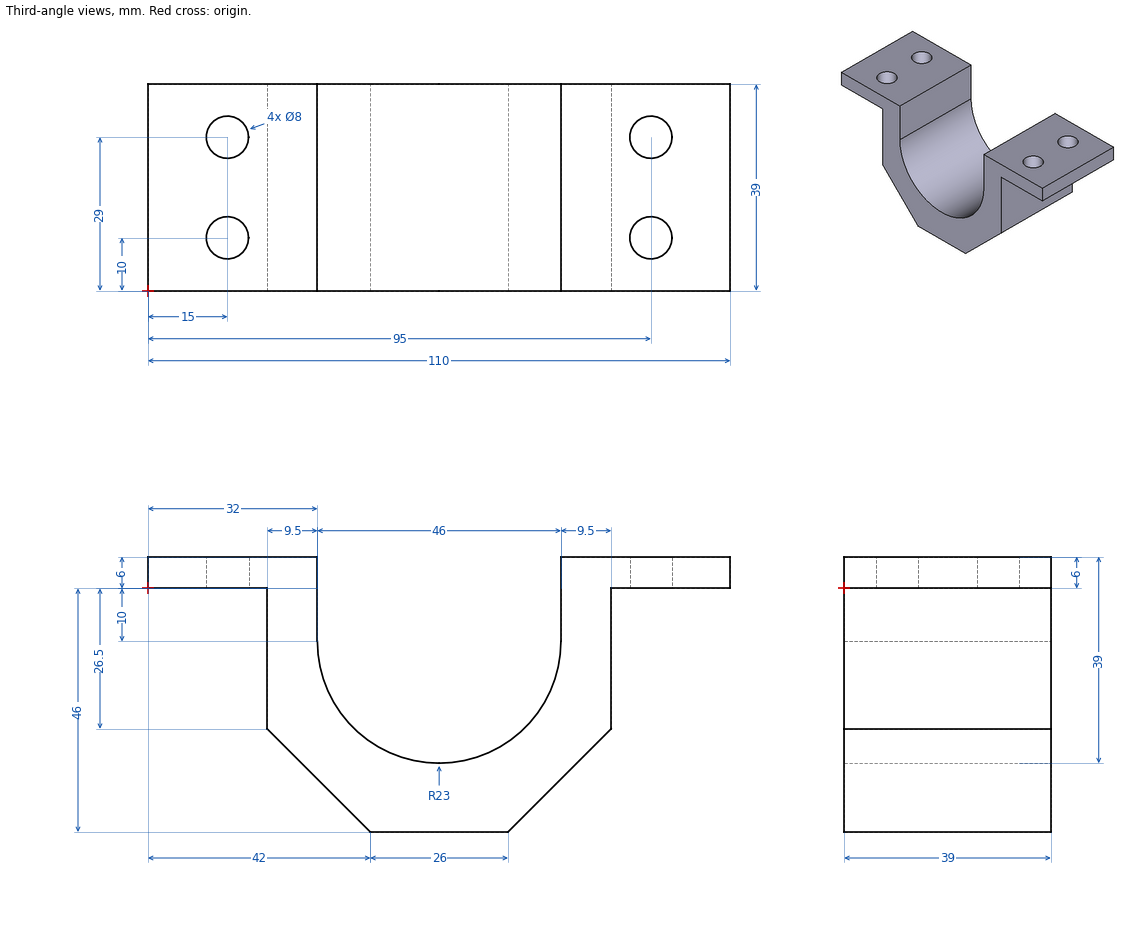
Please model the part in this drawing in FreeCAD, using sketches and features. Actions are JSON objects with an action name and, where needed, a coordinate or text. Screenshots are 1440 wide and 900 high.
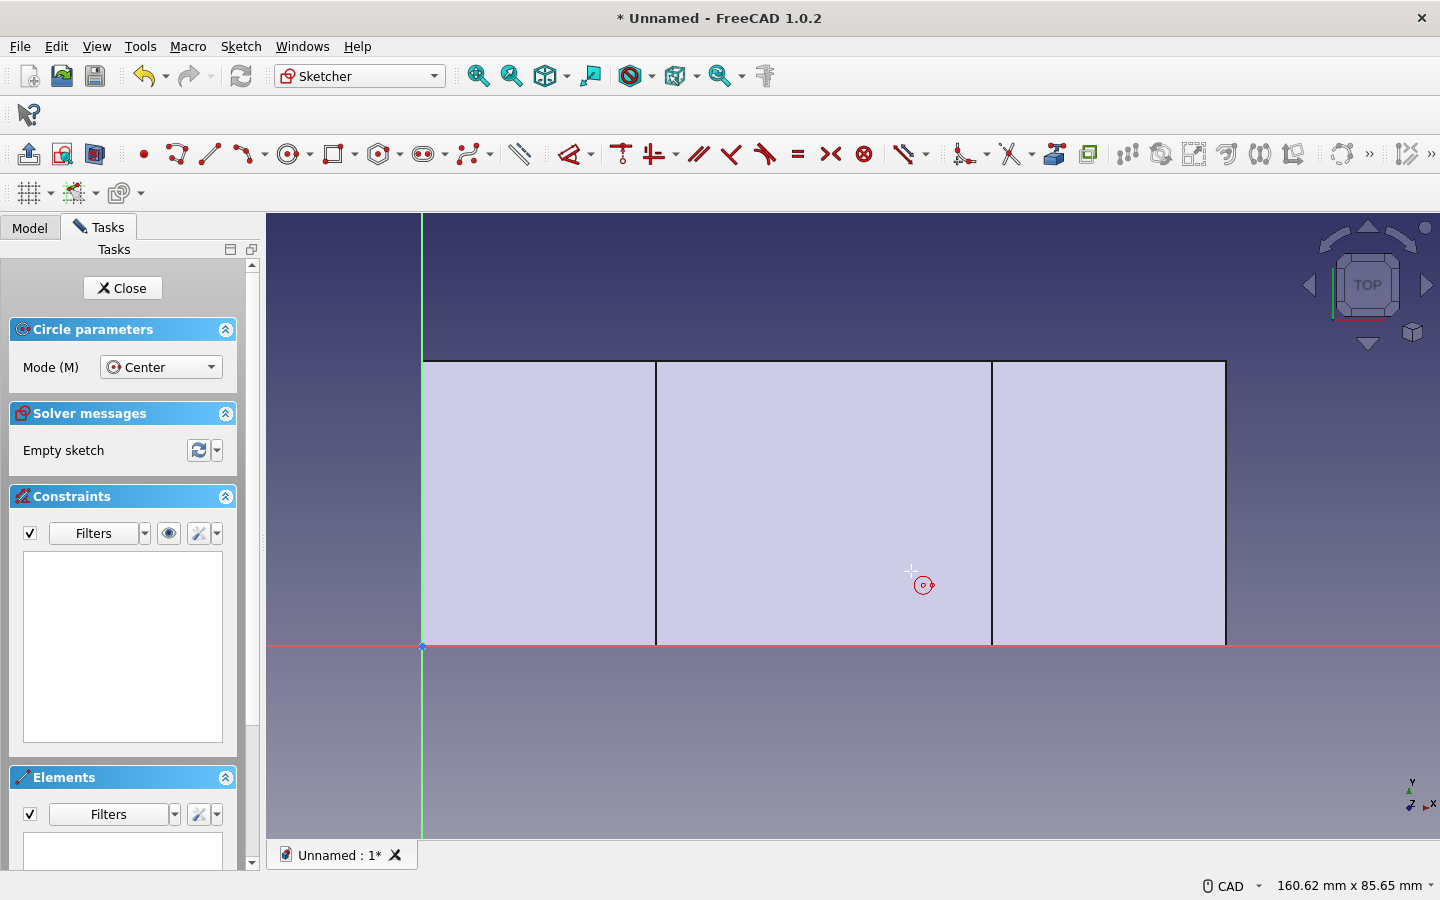
{"action": "left_click", "coordinate": [532, 434]}
{"action": "left_click", "coordinate": [553, 413]}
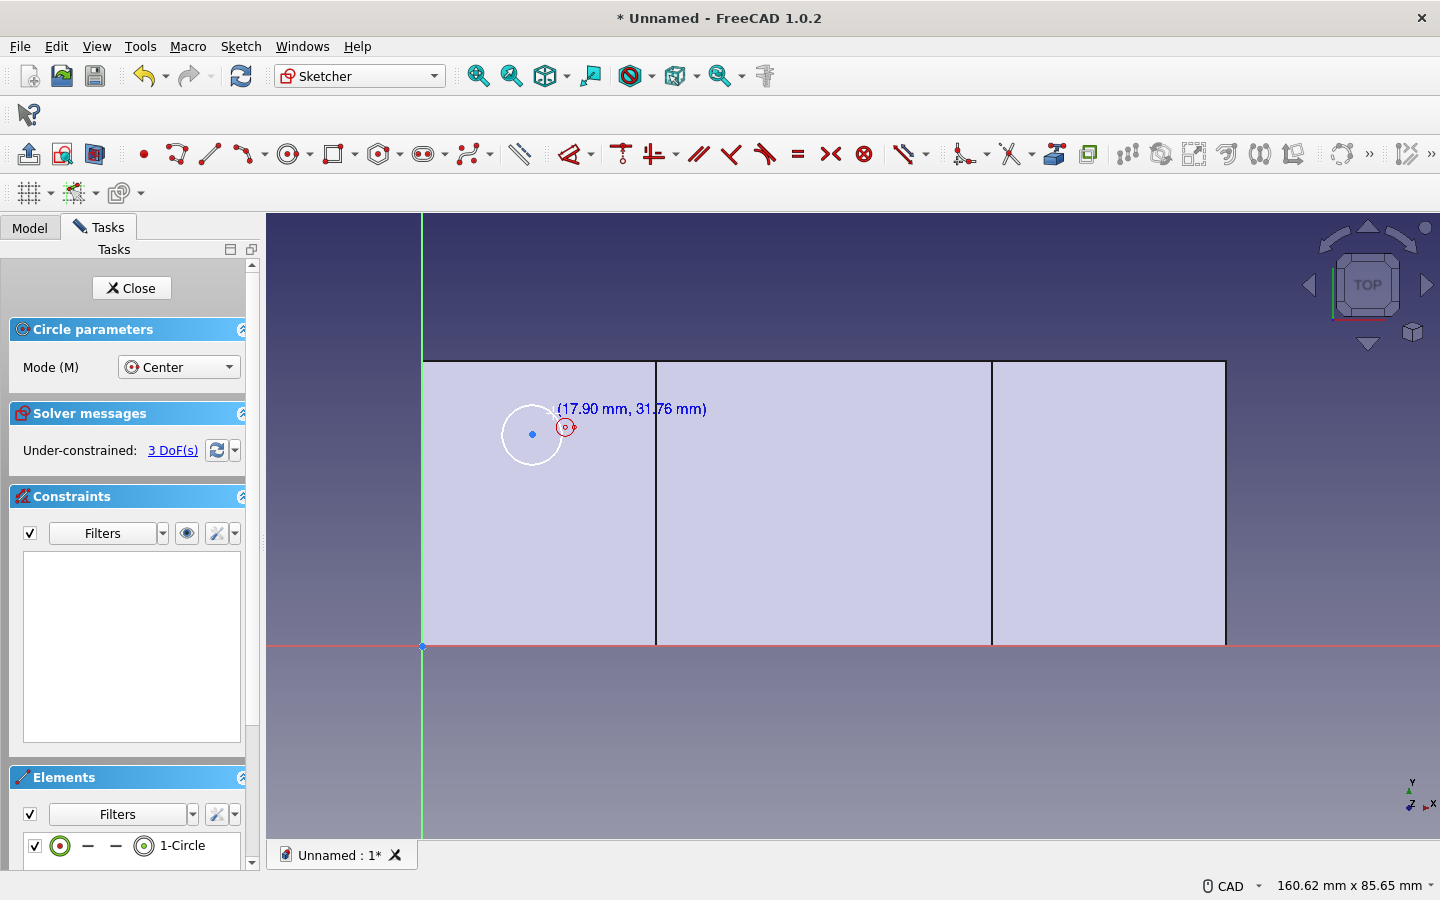
{"action": "left_click", "coordinate": [532, 573]}
{"action": "left_click", "coordinate": [553, 552]}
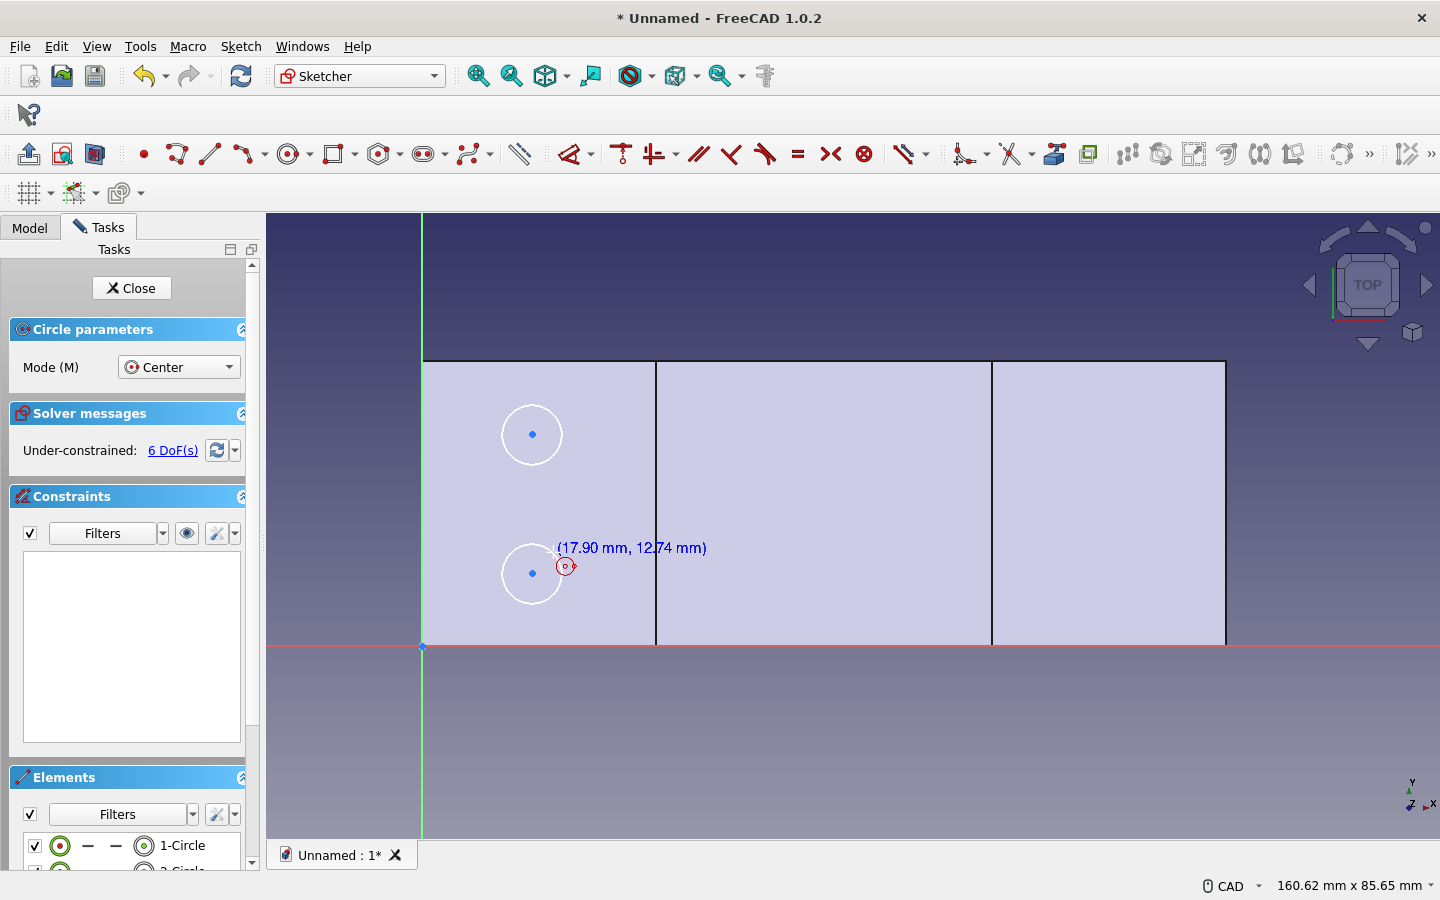
{"action": "left_click", "coordinate": [1117, 434]}
{"action": "left_click", "coordinate": [1137, 413]}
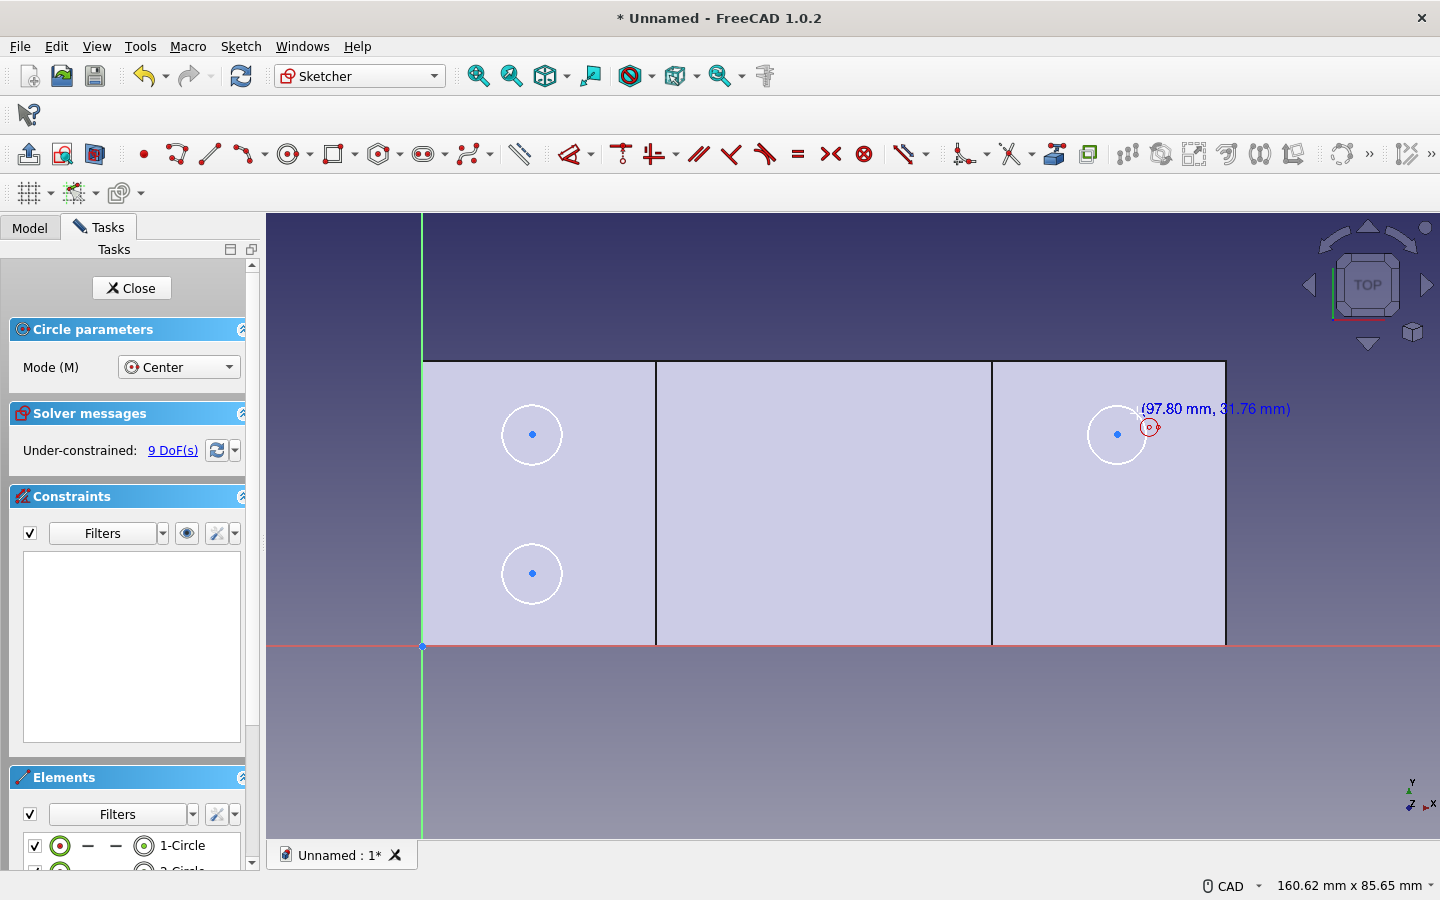
{"action": "left_click", "coordinate": [1117, 573]}
{"action": "left_click", "coordinate": [1137, 552]}
{"action": "key", "text": "Escape"}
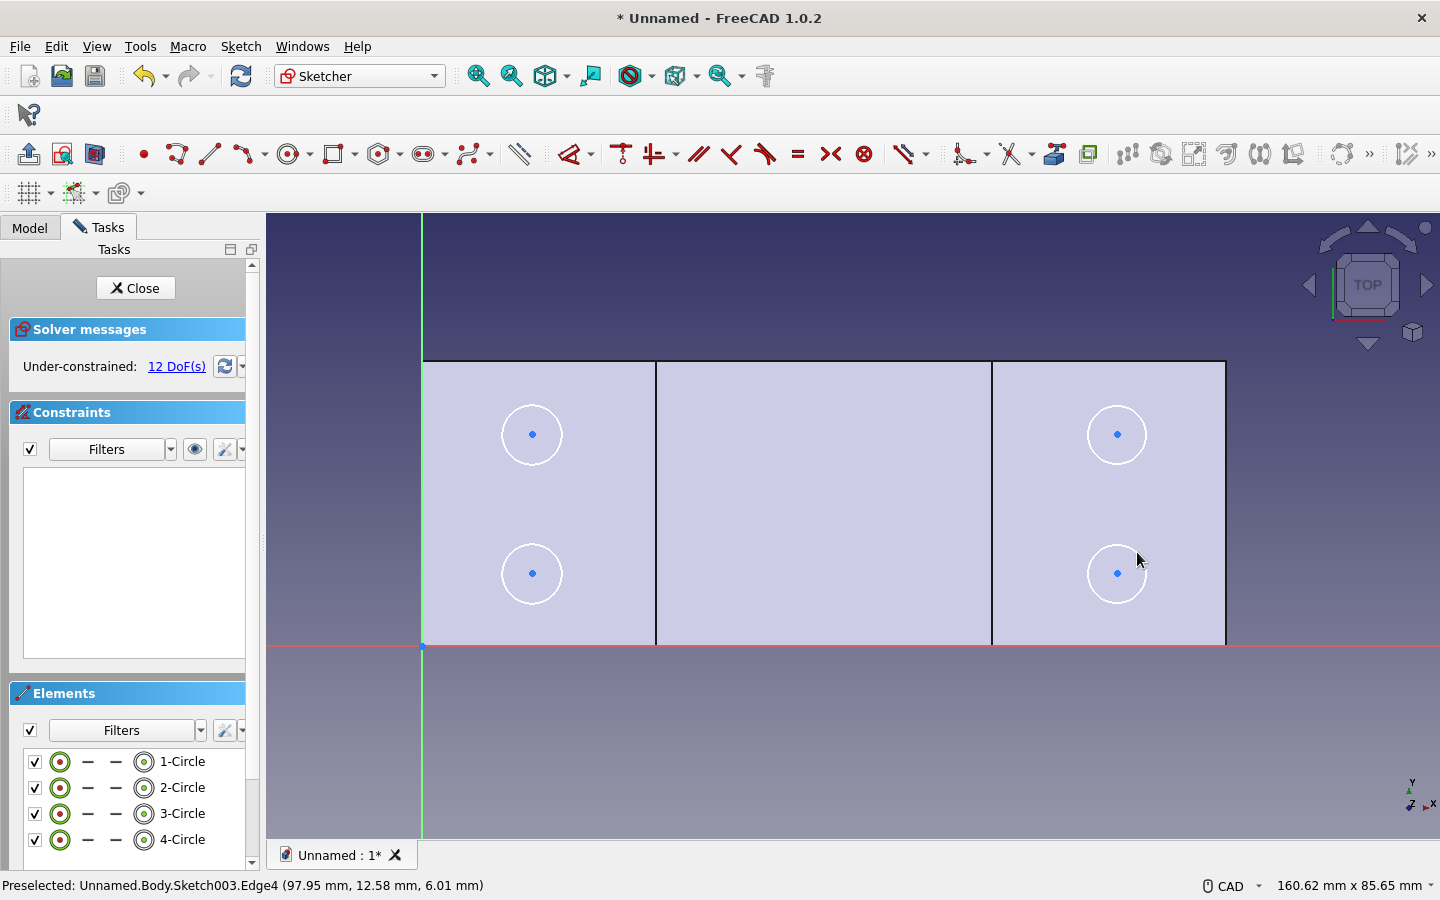
{"action": "left_click", "coordinate": [553, 414]}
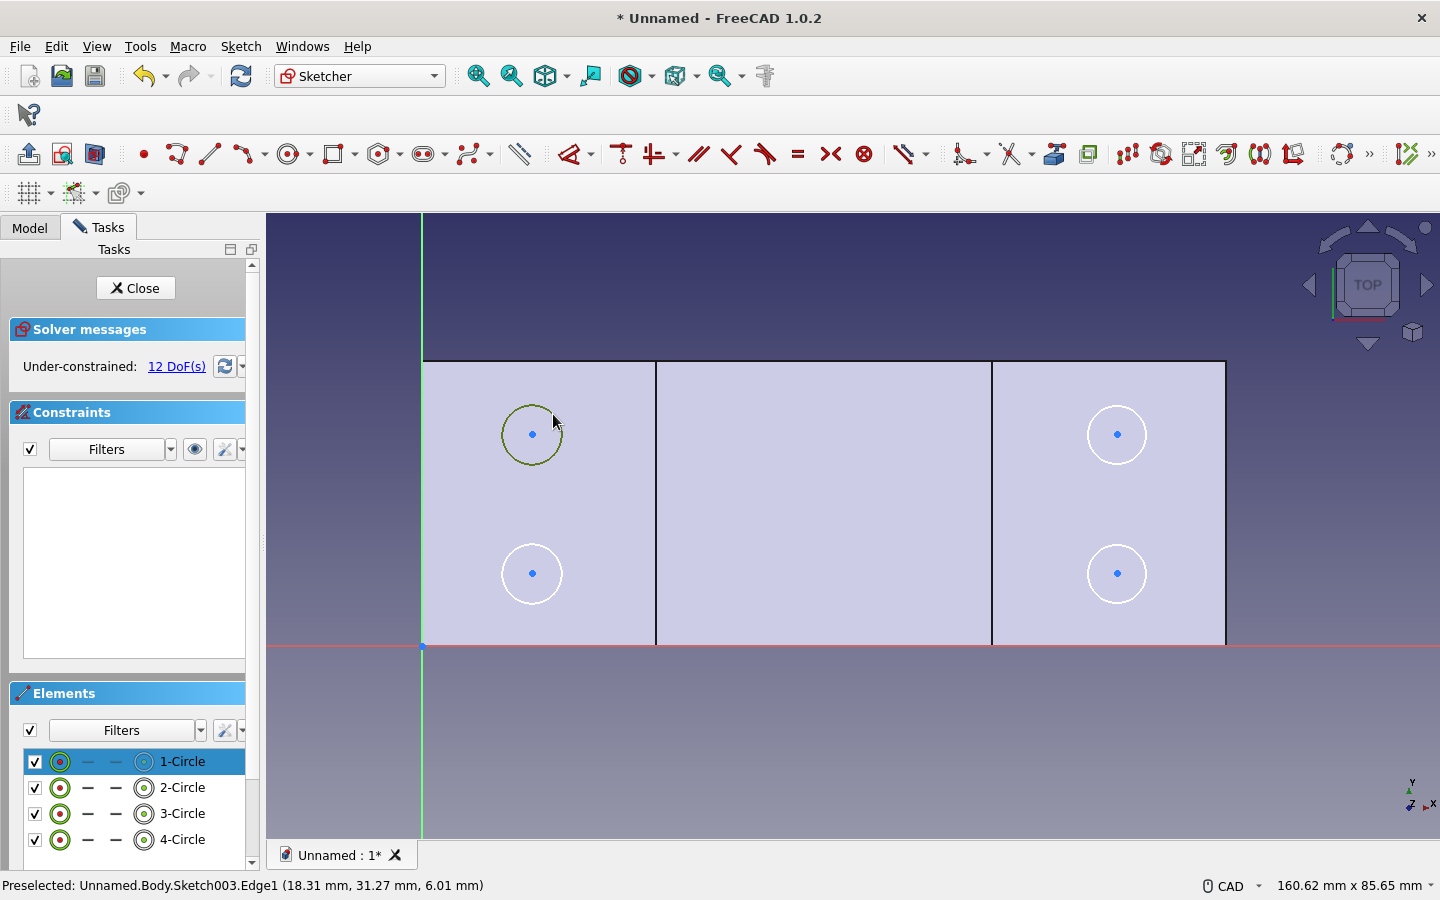
{"action": "left_click", "coordinate": [553, 553]}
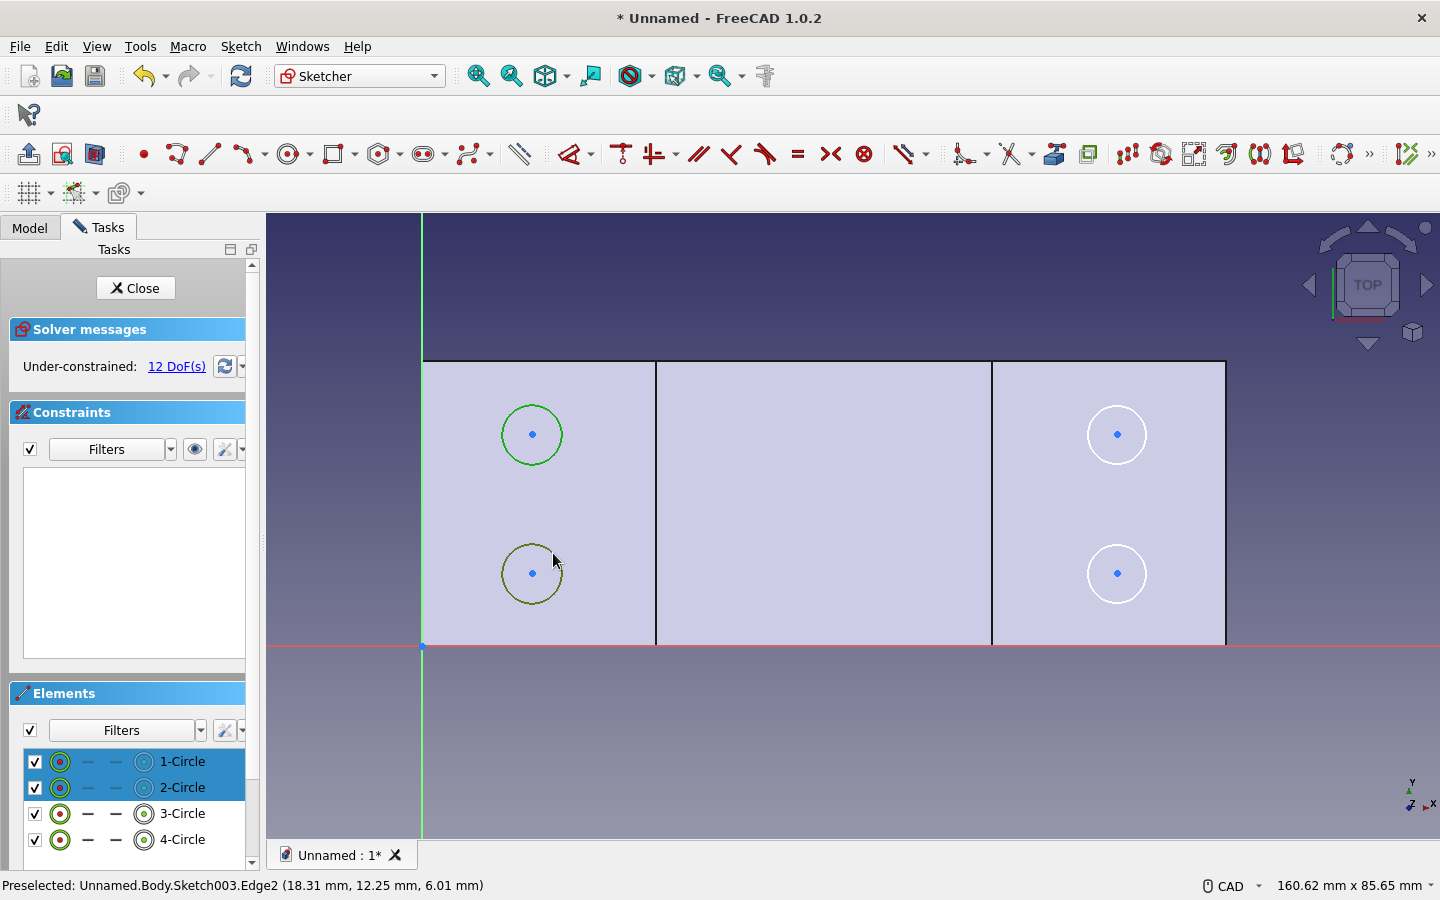
{"action": "left_click", "coordinate": [1137, 414]}